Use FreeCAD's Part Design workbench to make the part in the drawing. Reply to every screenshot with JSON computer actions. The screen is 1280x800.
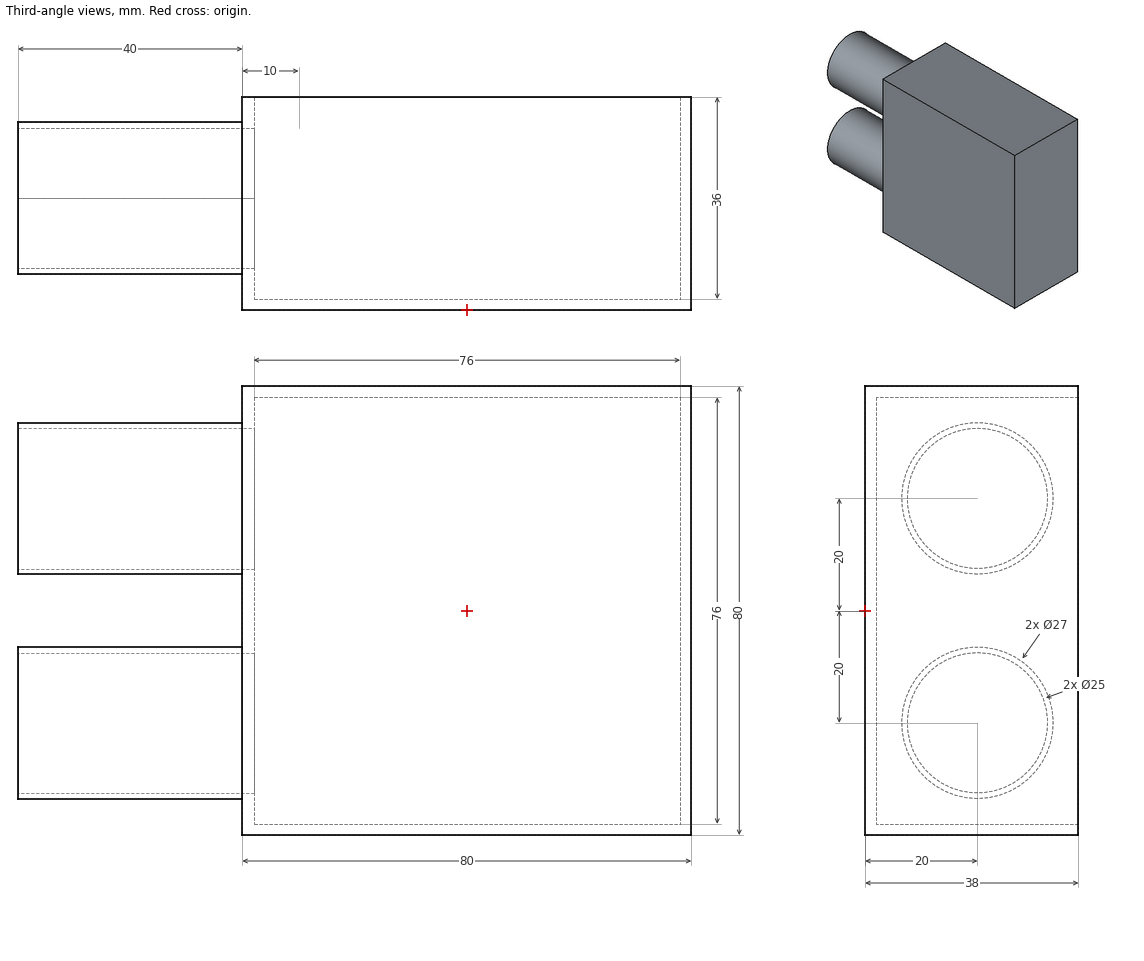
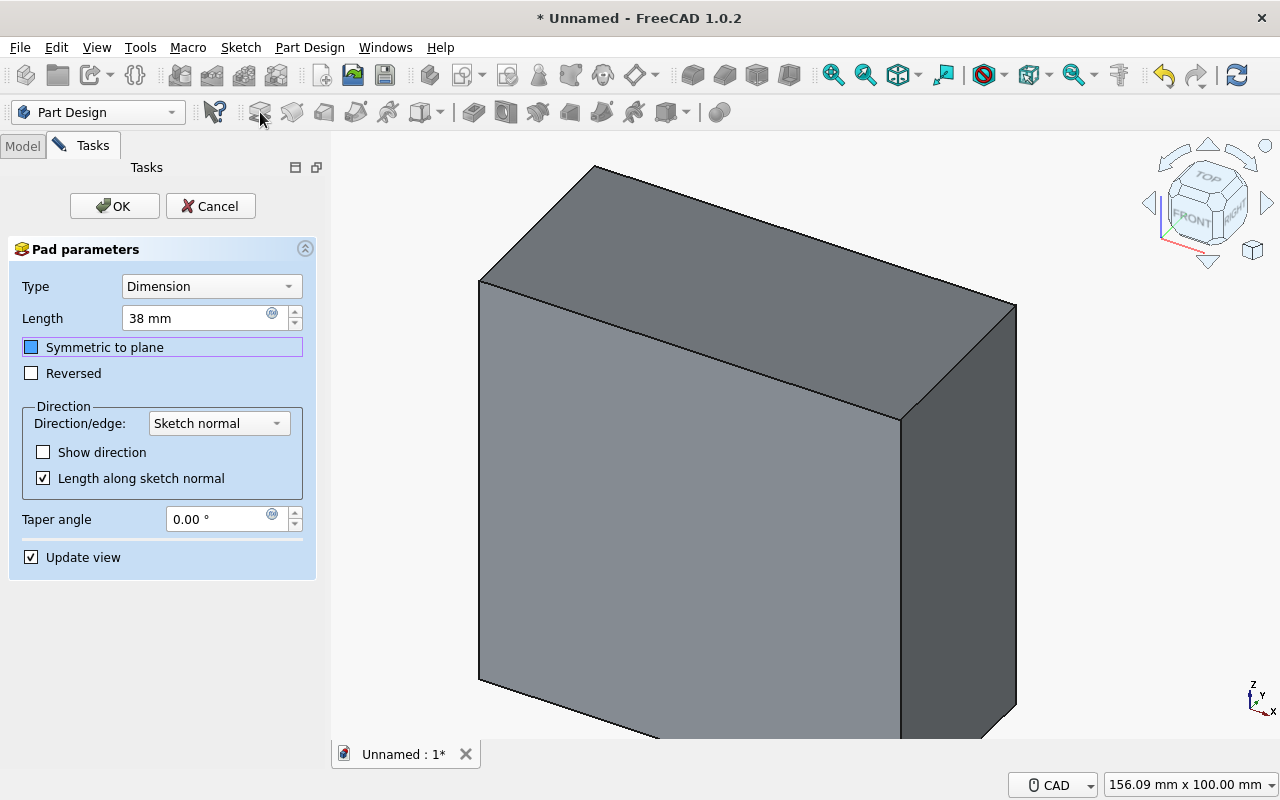
{"action": "left_click", "coordinate": [30, 373]}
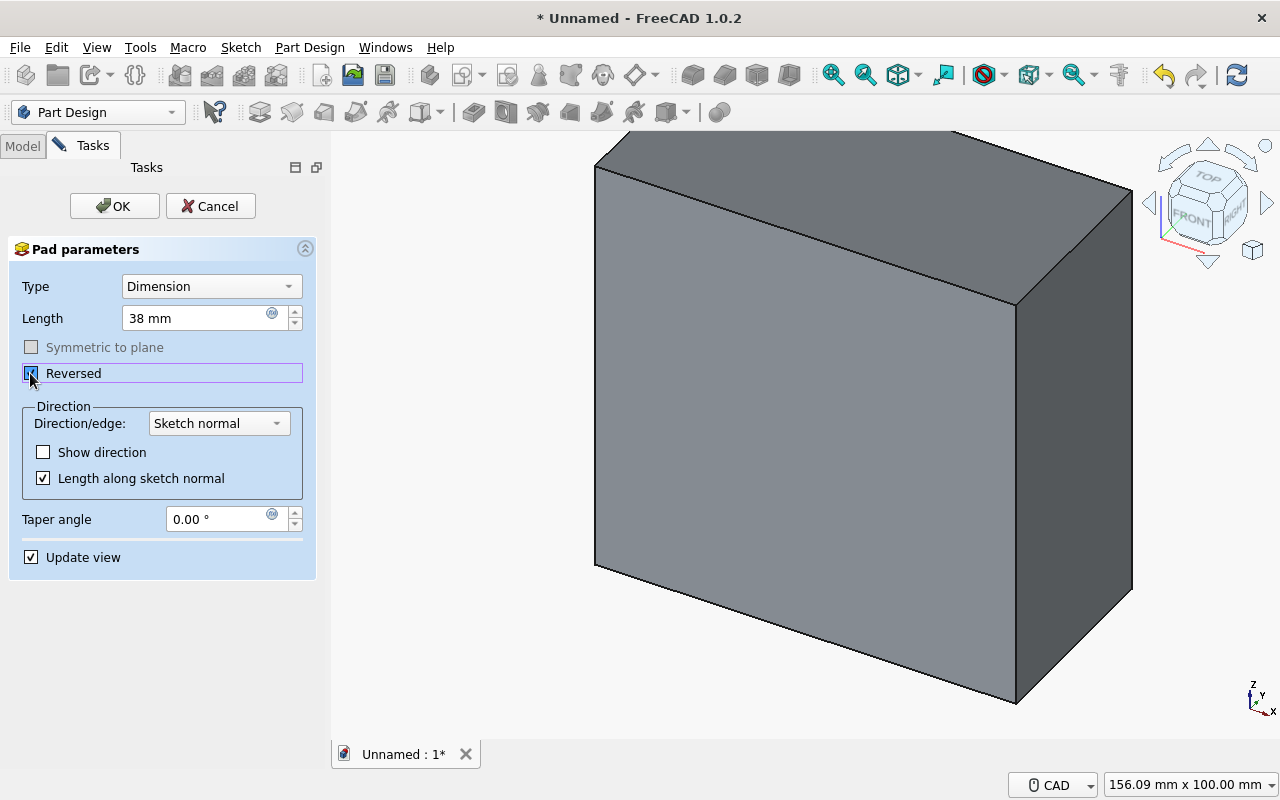
{"action": "left_click", "coordinate": [115, 206]}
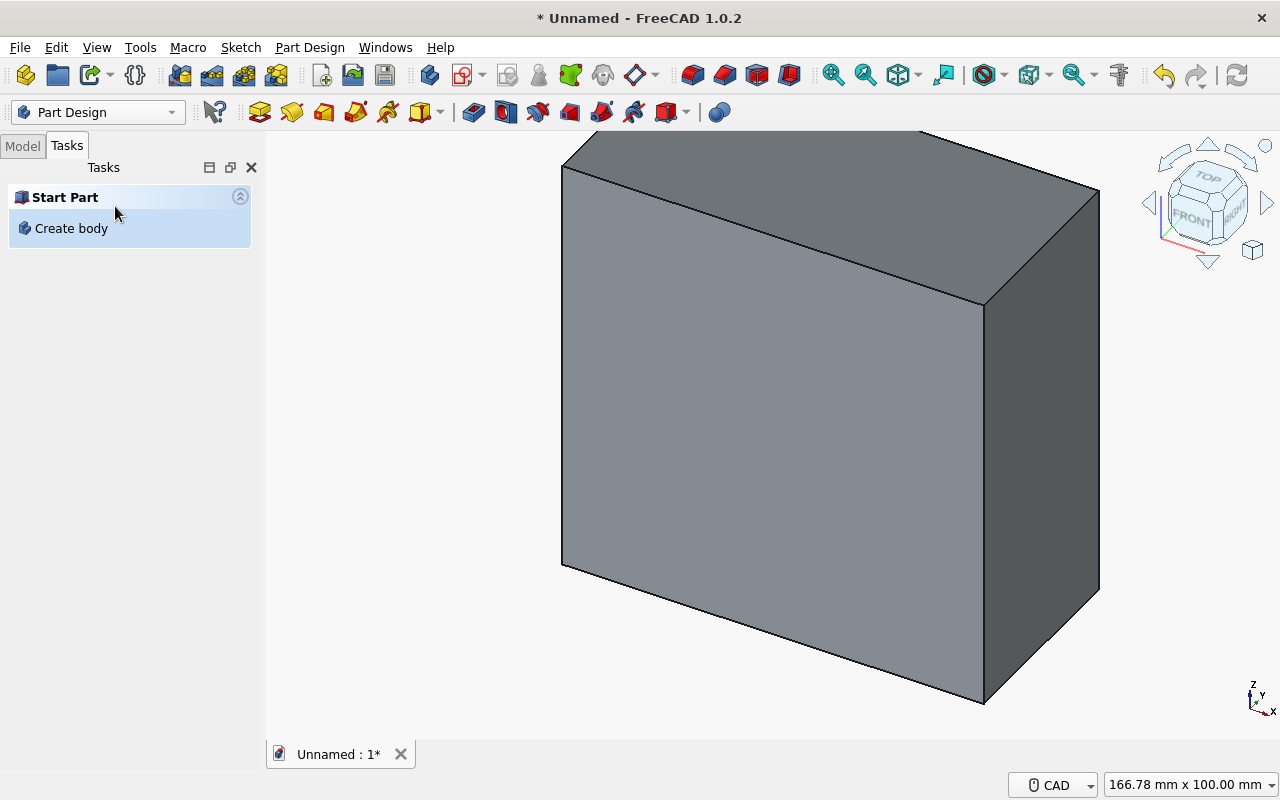
{"action": "left_click", "coordinate": [834, 76]}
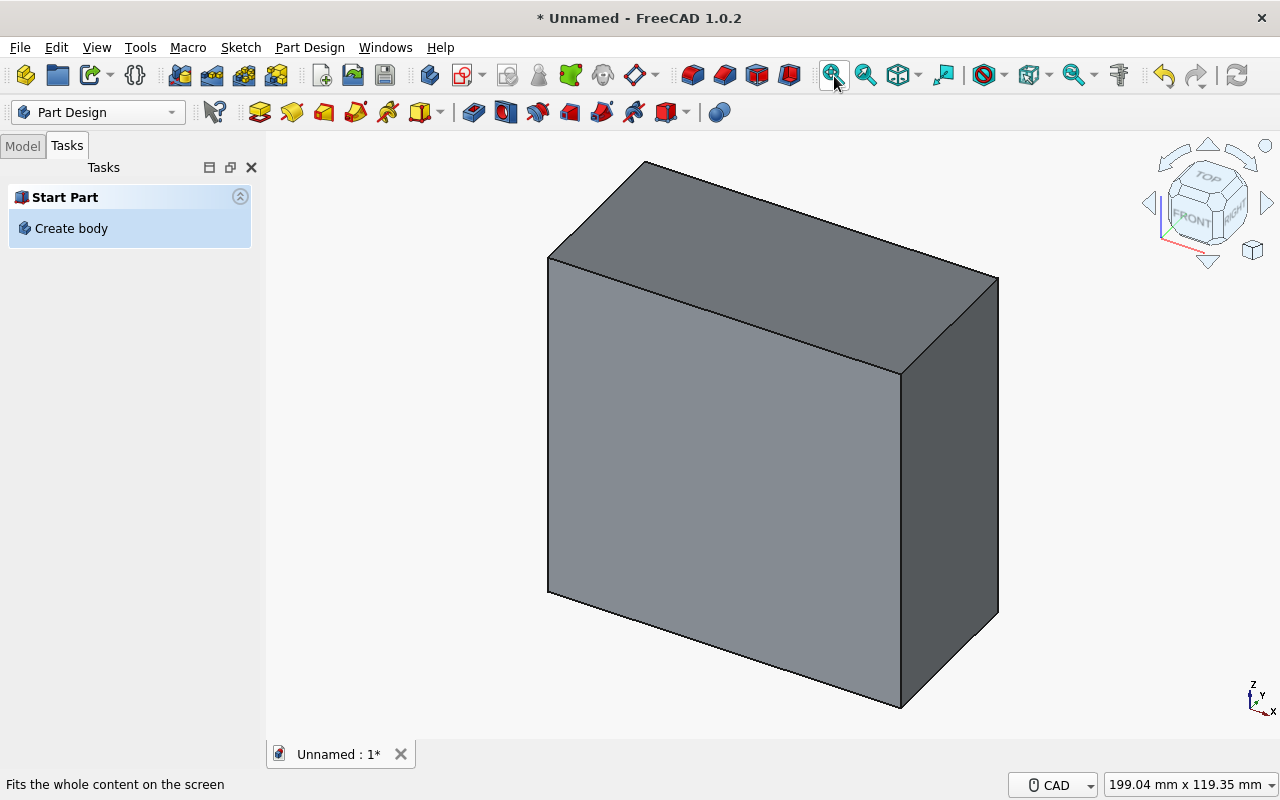
{"action": "key", "text": "4"}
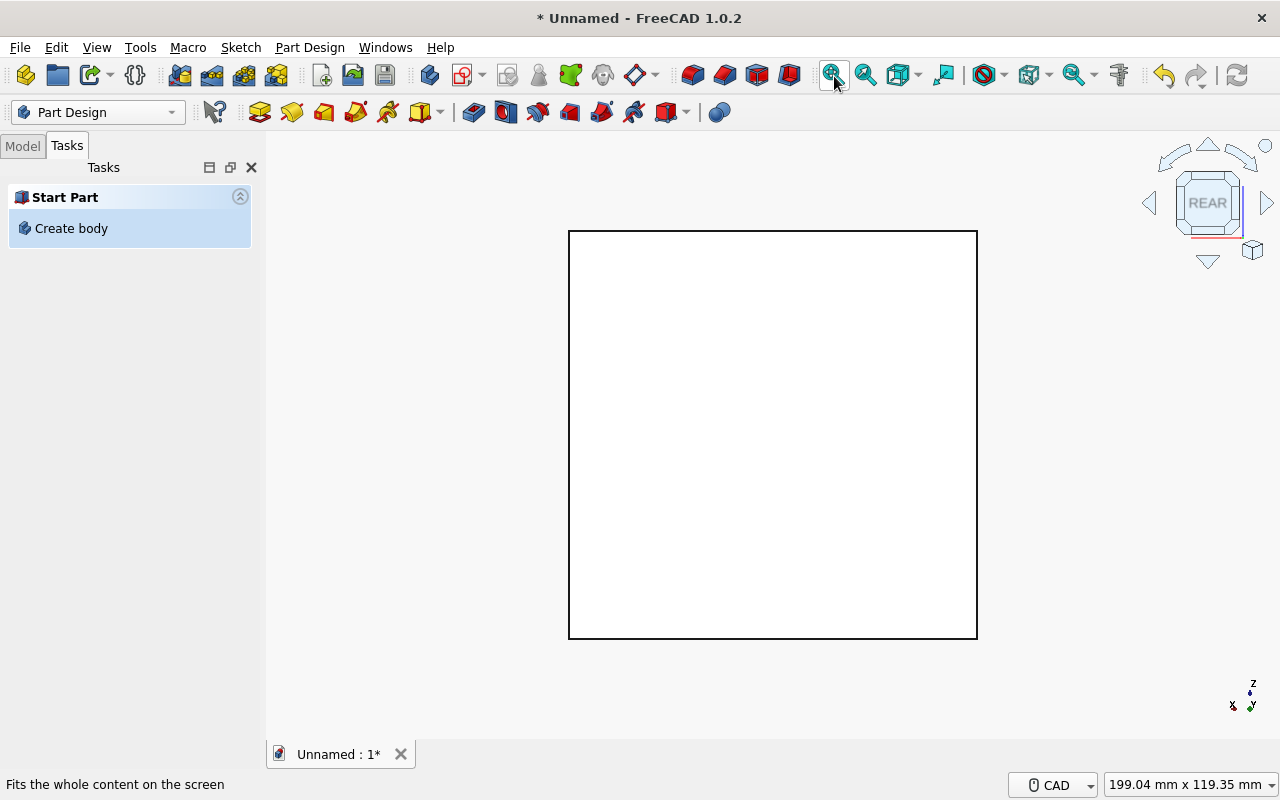
{"action": "left_click", "coordinate": [773, 434]}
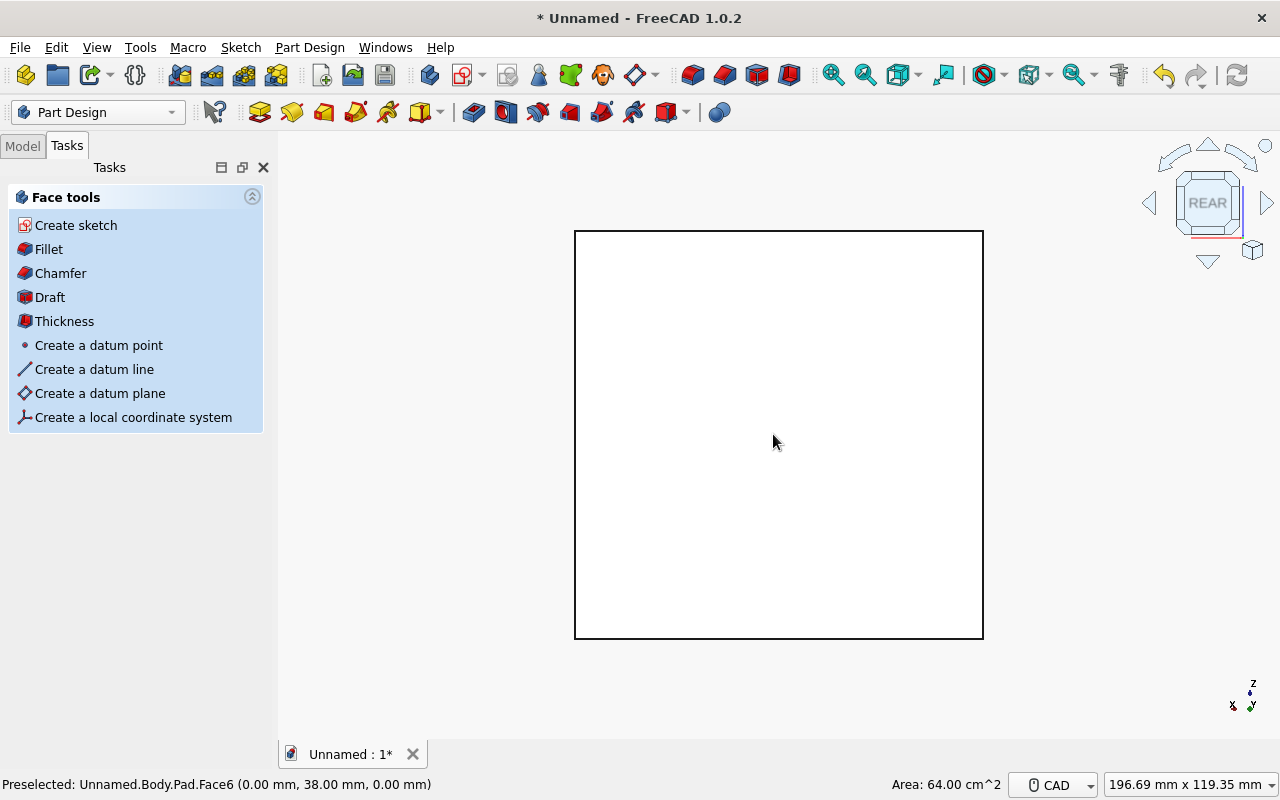
{"action": "left_click", "coordinate": [462, 76]}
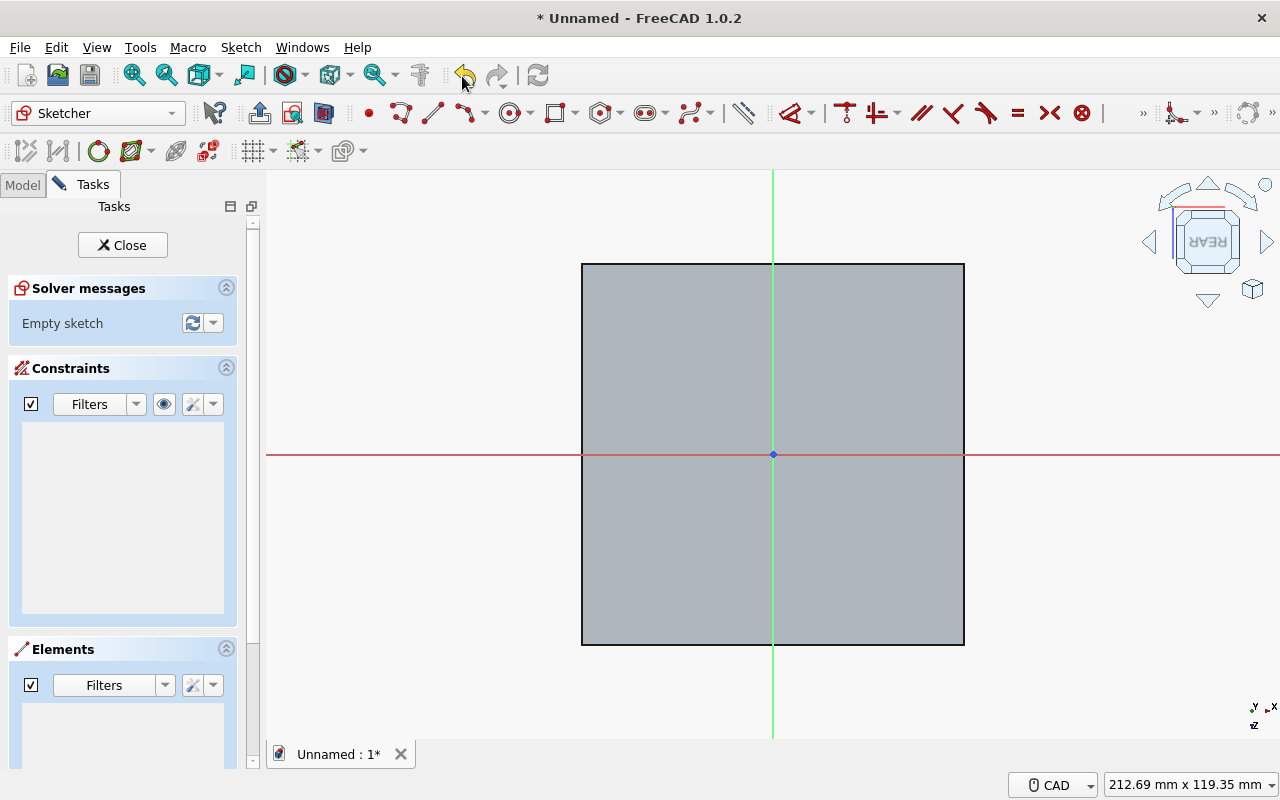
{"action": "key", "text": "g v"}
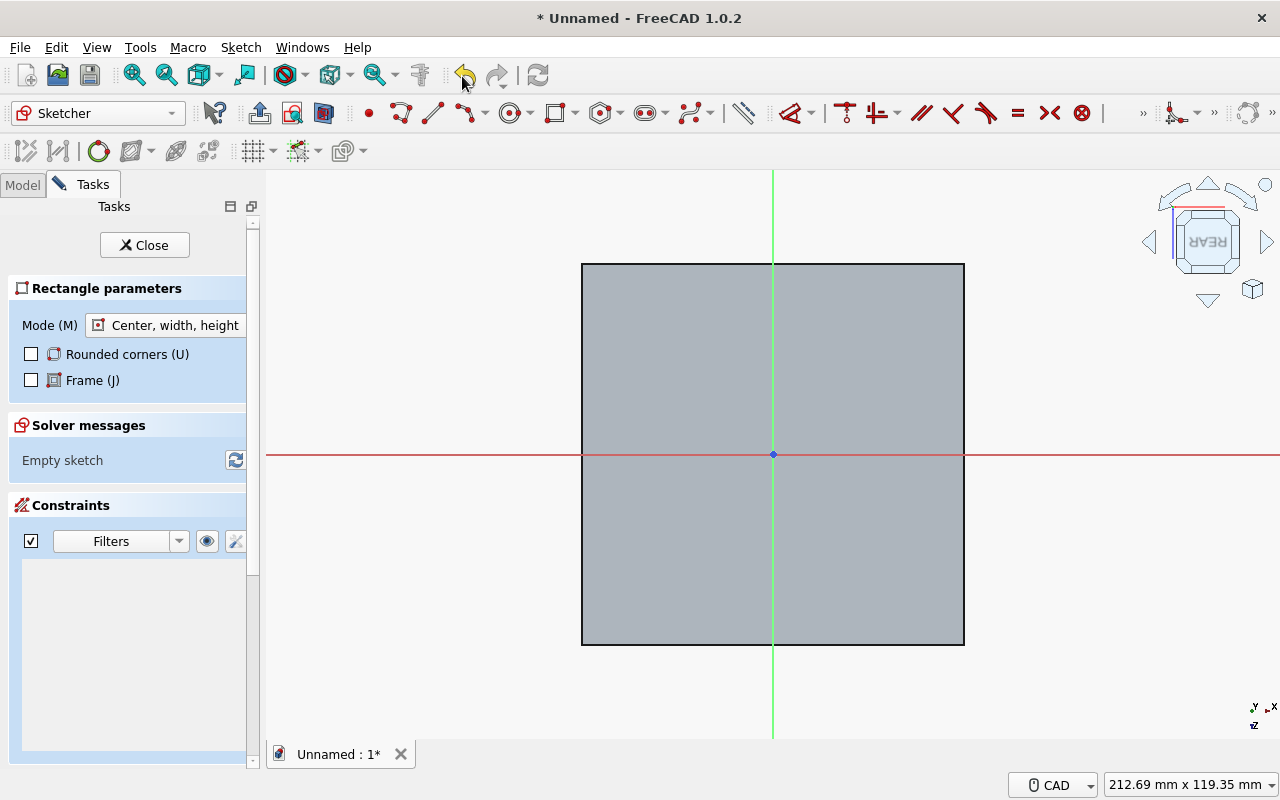
{"action": "left_click", "coordinate": [773, 455]}
{"action": "mouse_move", "coordinate": [954, 273]}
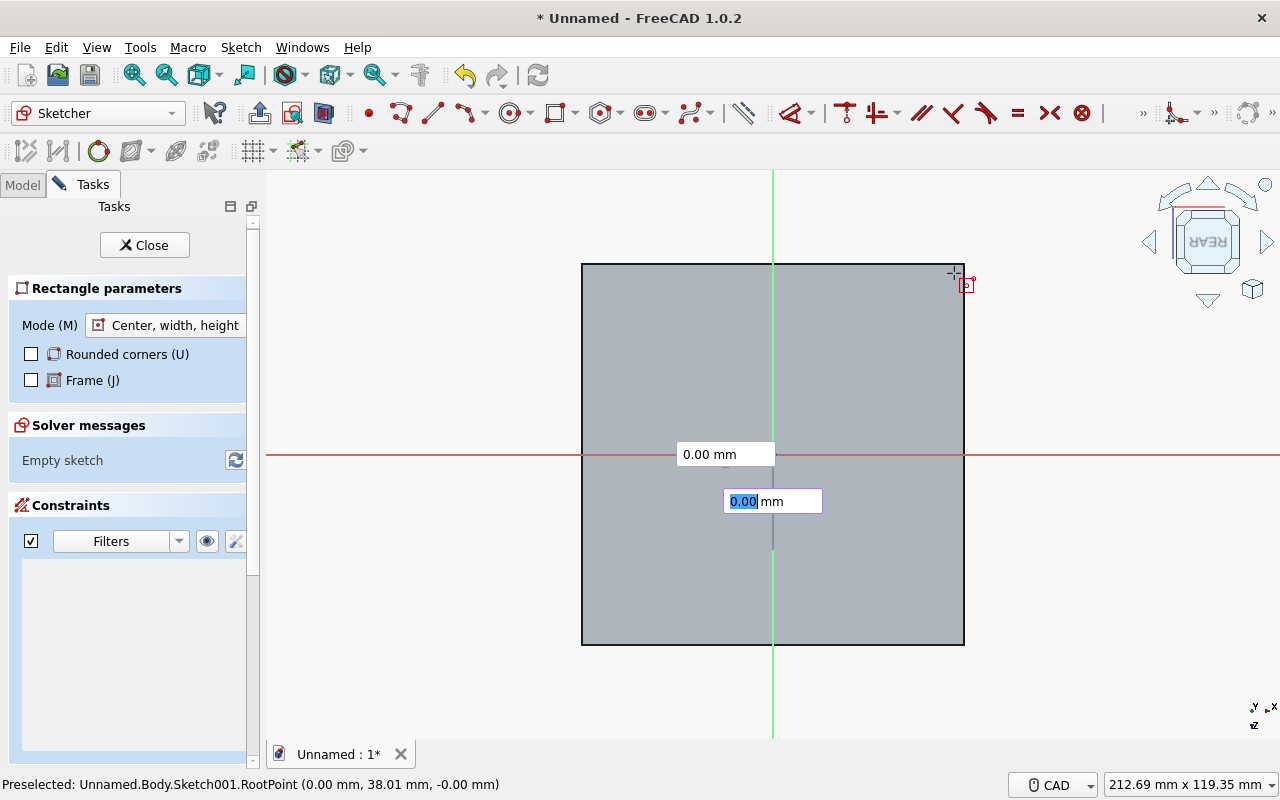
{"action": "type", "text": "76"}
{"action": "key", "text": "Tab"}
{"action": "type", "text": "76"}
{"action": "key", "text": "Return"}
{"action": "key", "text": "Escape"}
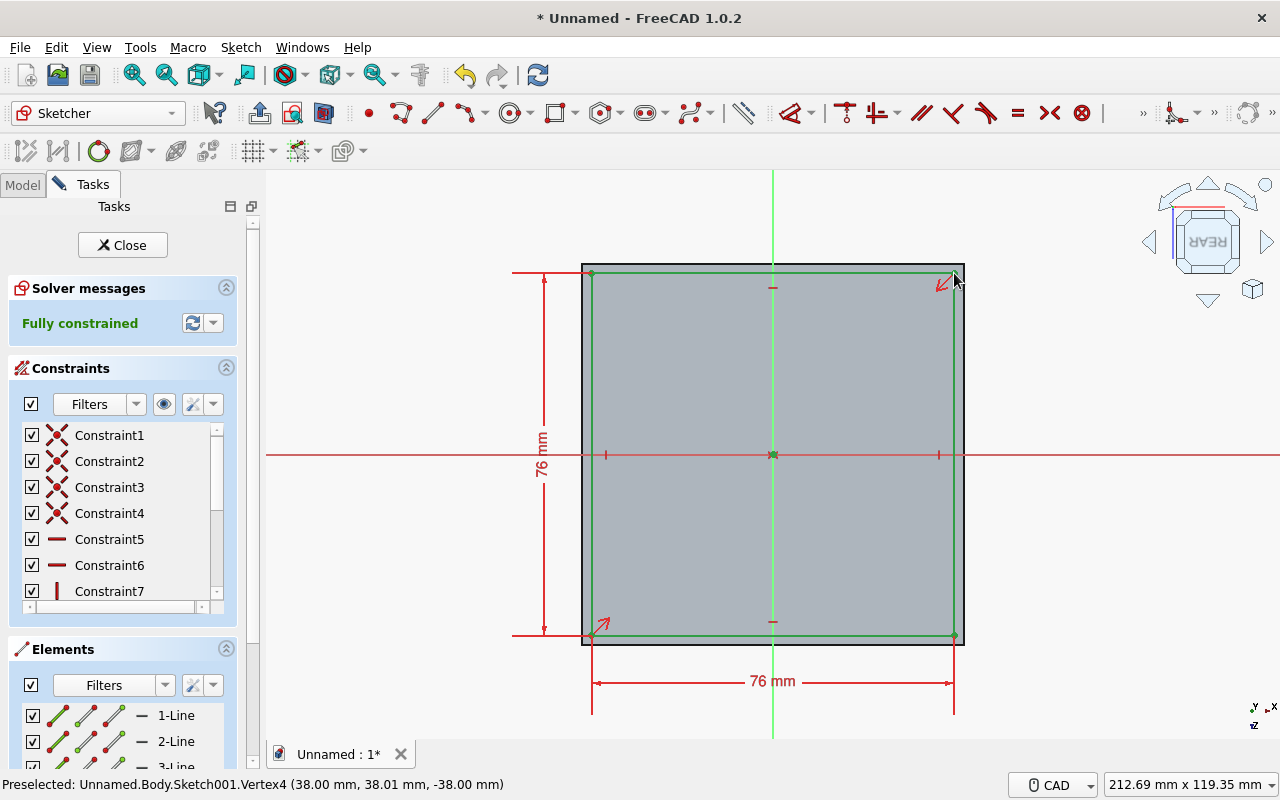
{"action": "left_click", "coordinate": [123, 245]}